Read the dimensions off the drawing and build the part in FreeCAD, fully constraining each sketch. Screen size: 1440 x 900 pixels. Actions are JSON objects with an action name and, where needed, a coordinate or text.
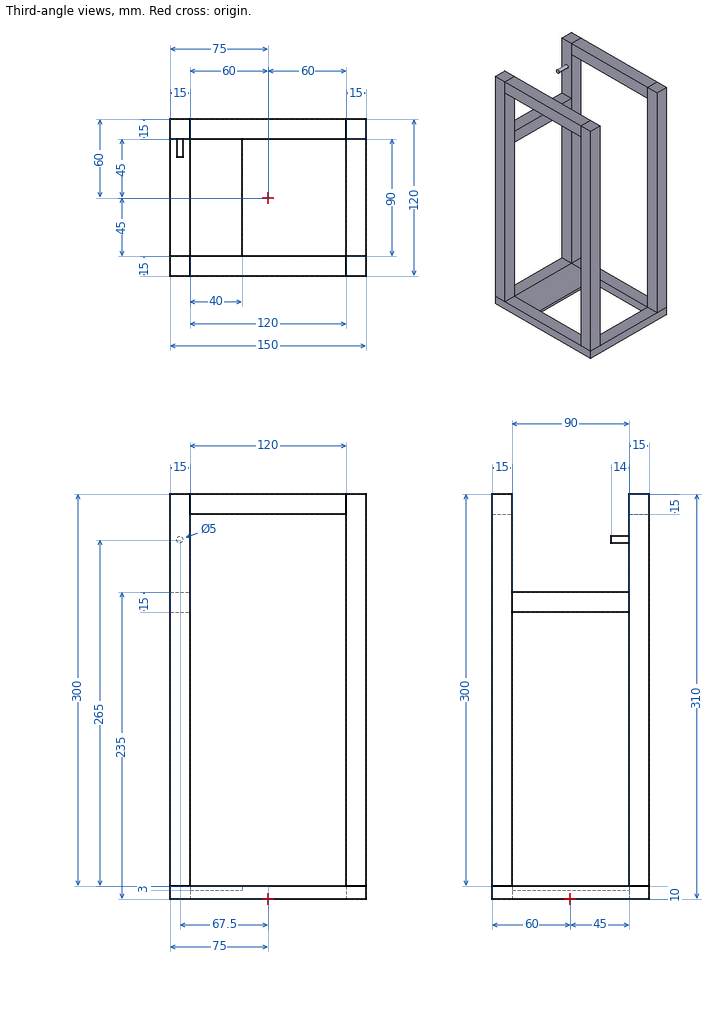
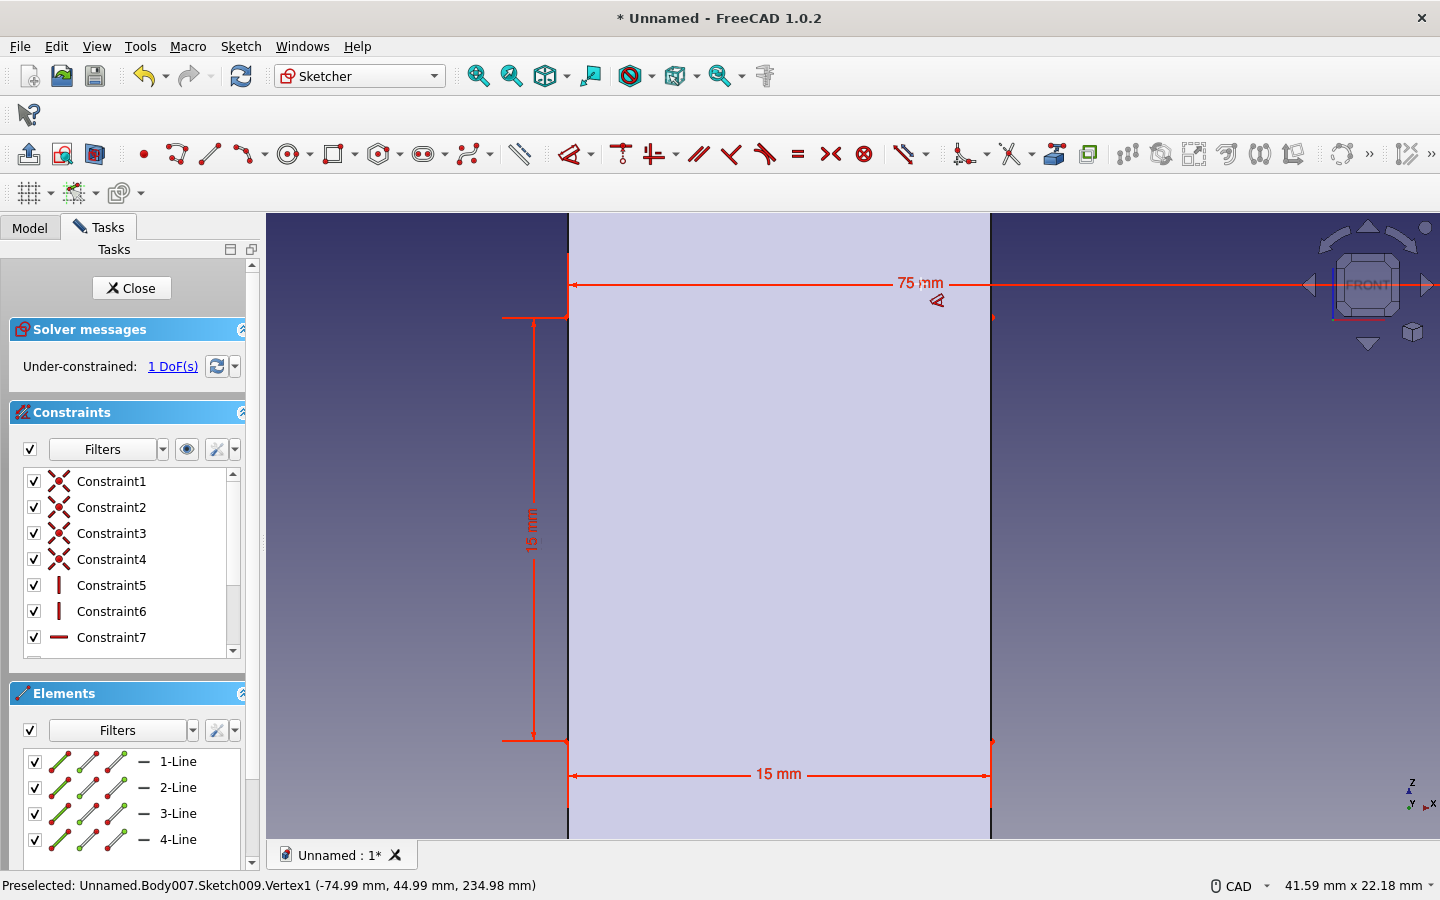
{"action": "left_click", "coordinate": [568, 318]}
{"action": "left_click", "coordinate": [534, 564]}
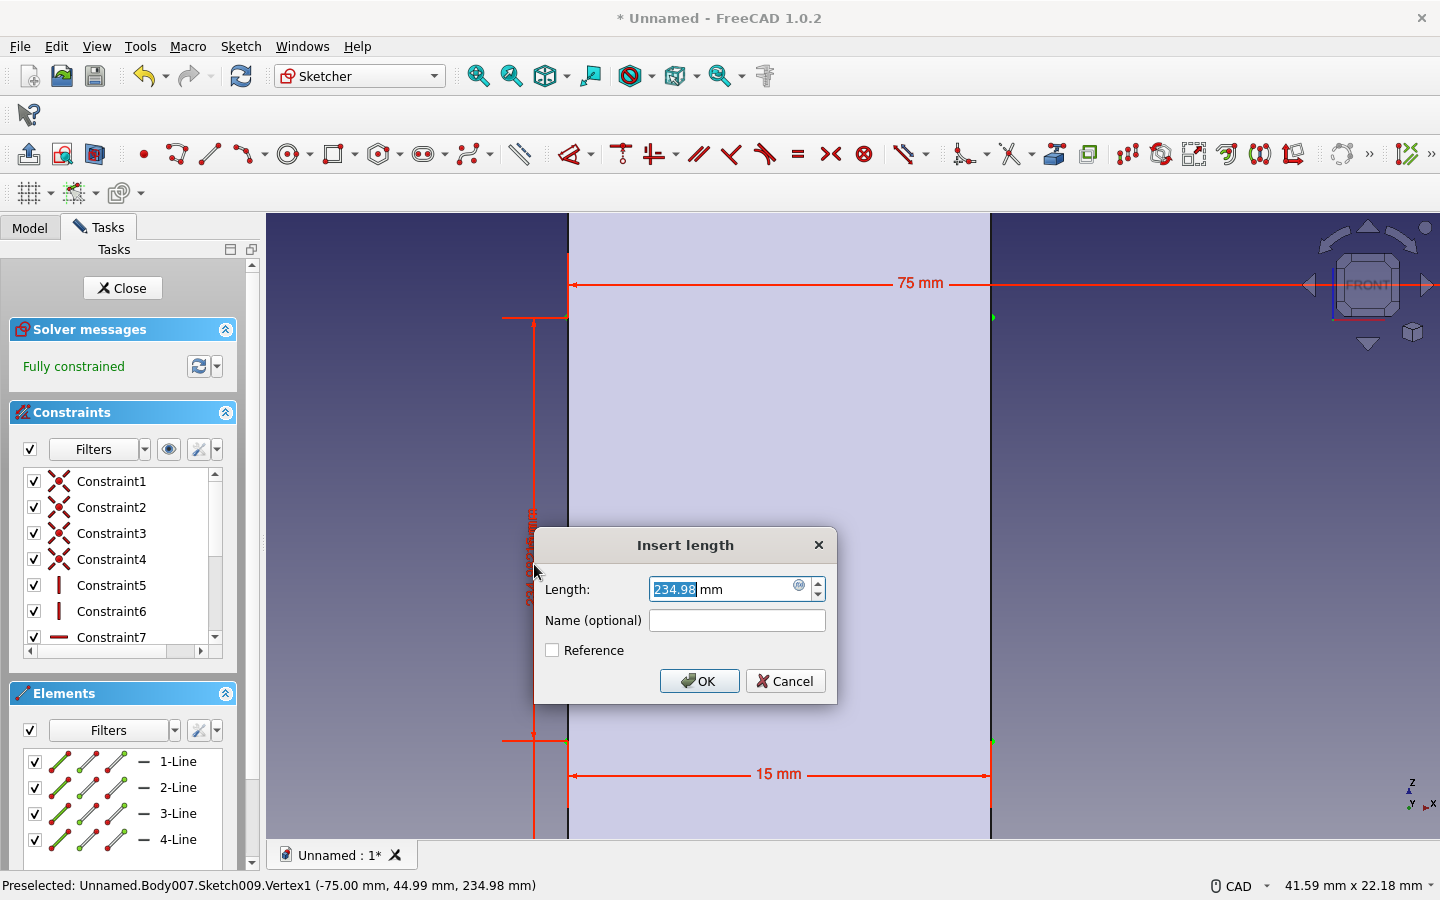
{"action": "type", "text": "235"}
{"action": "key", "text": "Return"}
{"action": "key", "text": "Escape"}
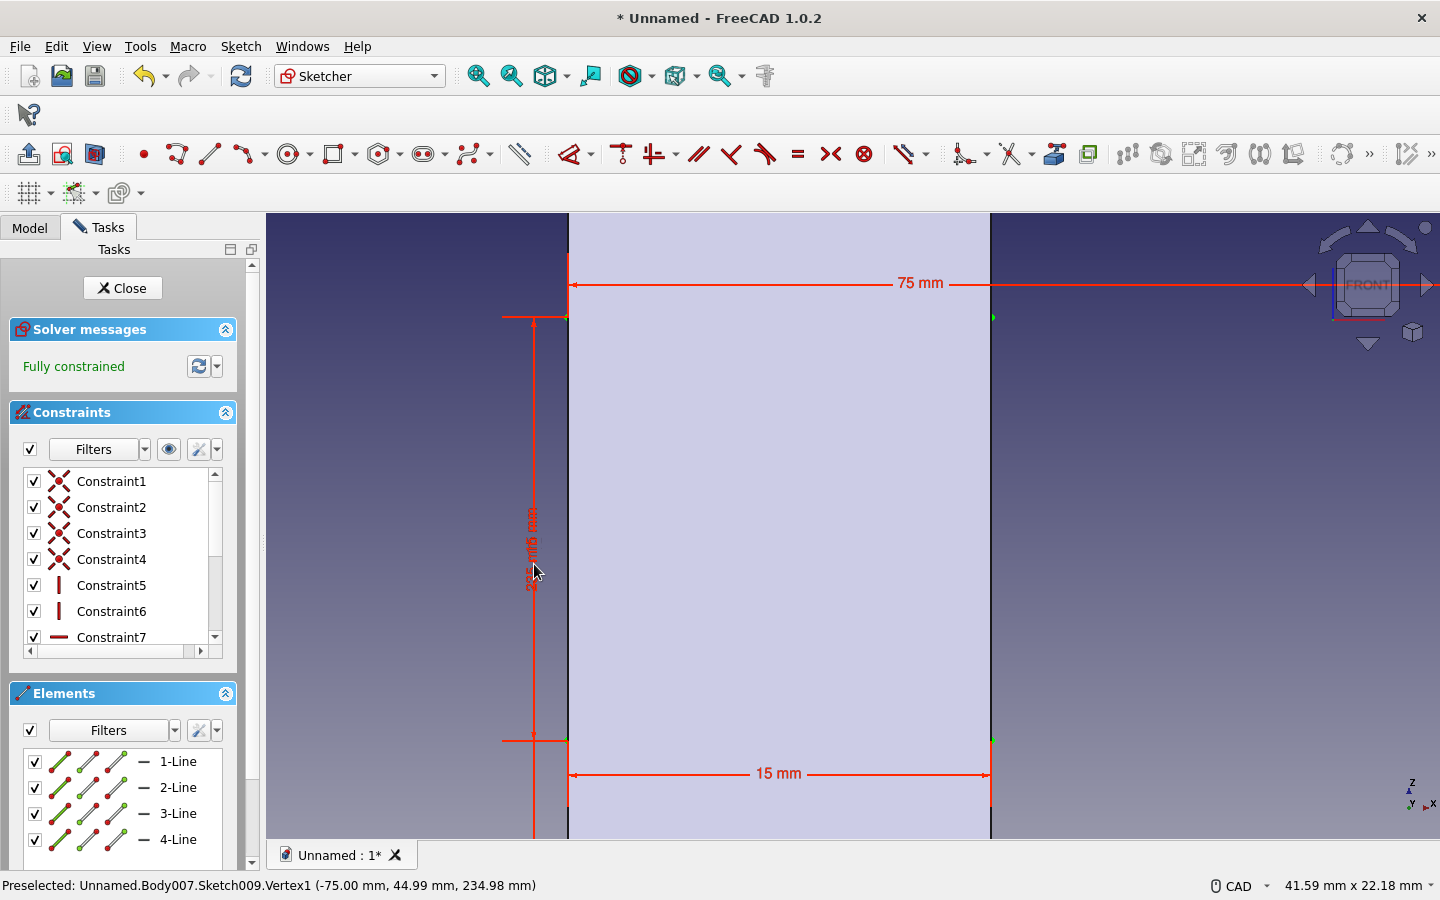
{"action": "left_click", "coordinate": [123, 288]}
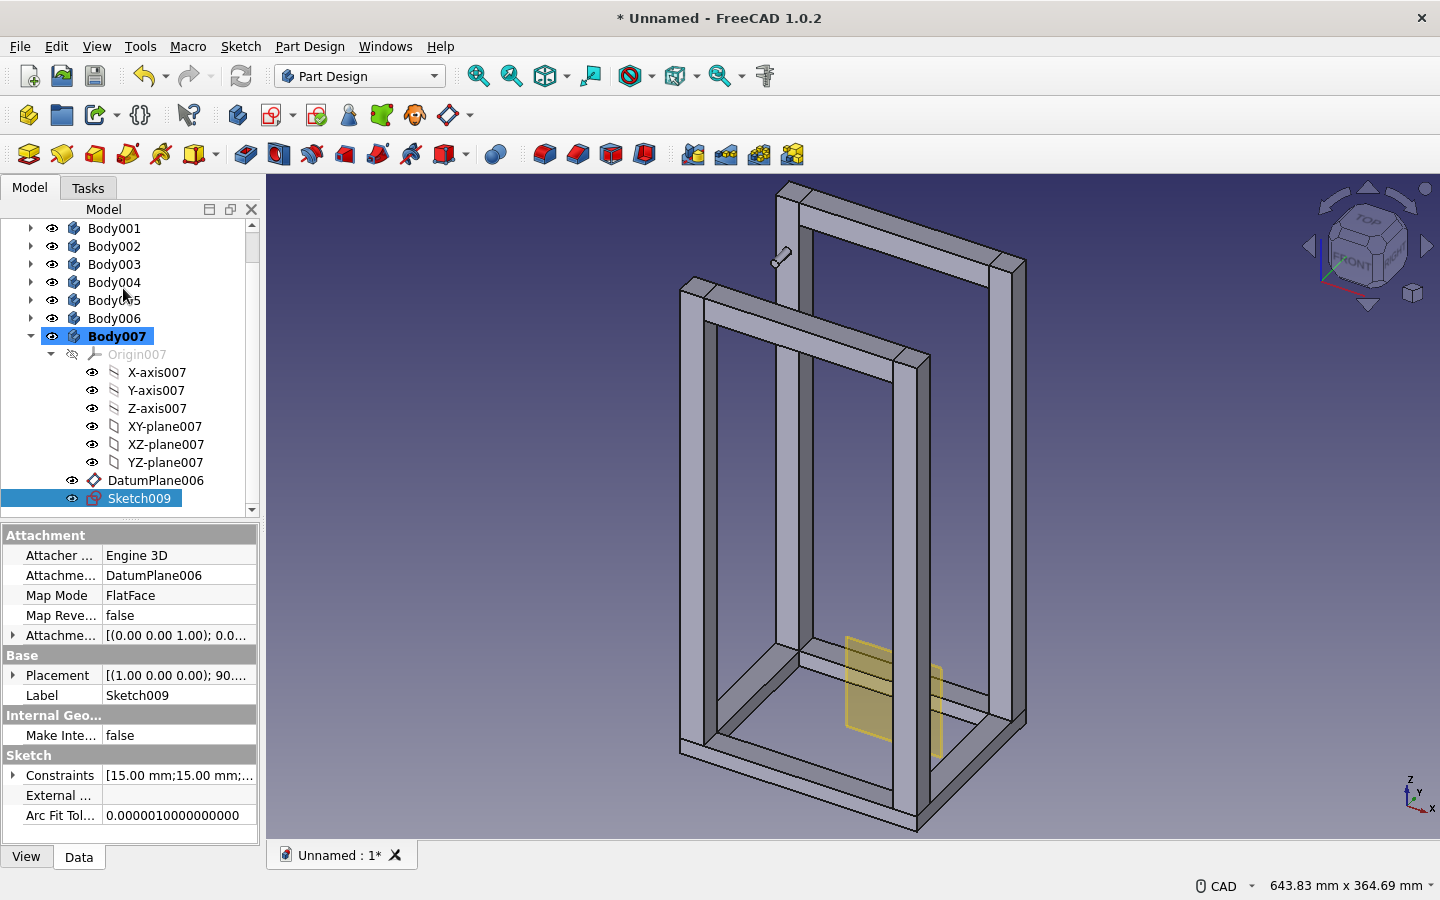
{"action": "left_click", "coordinate": [29, 154]}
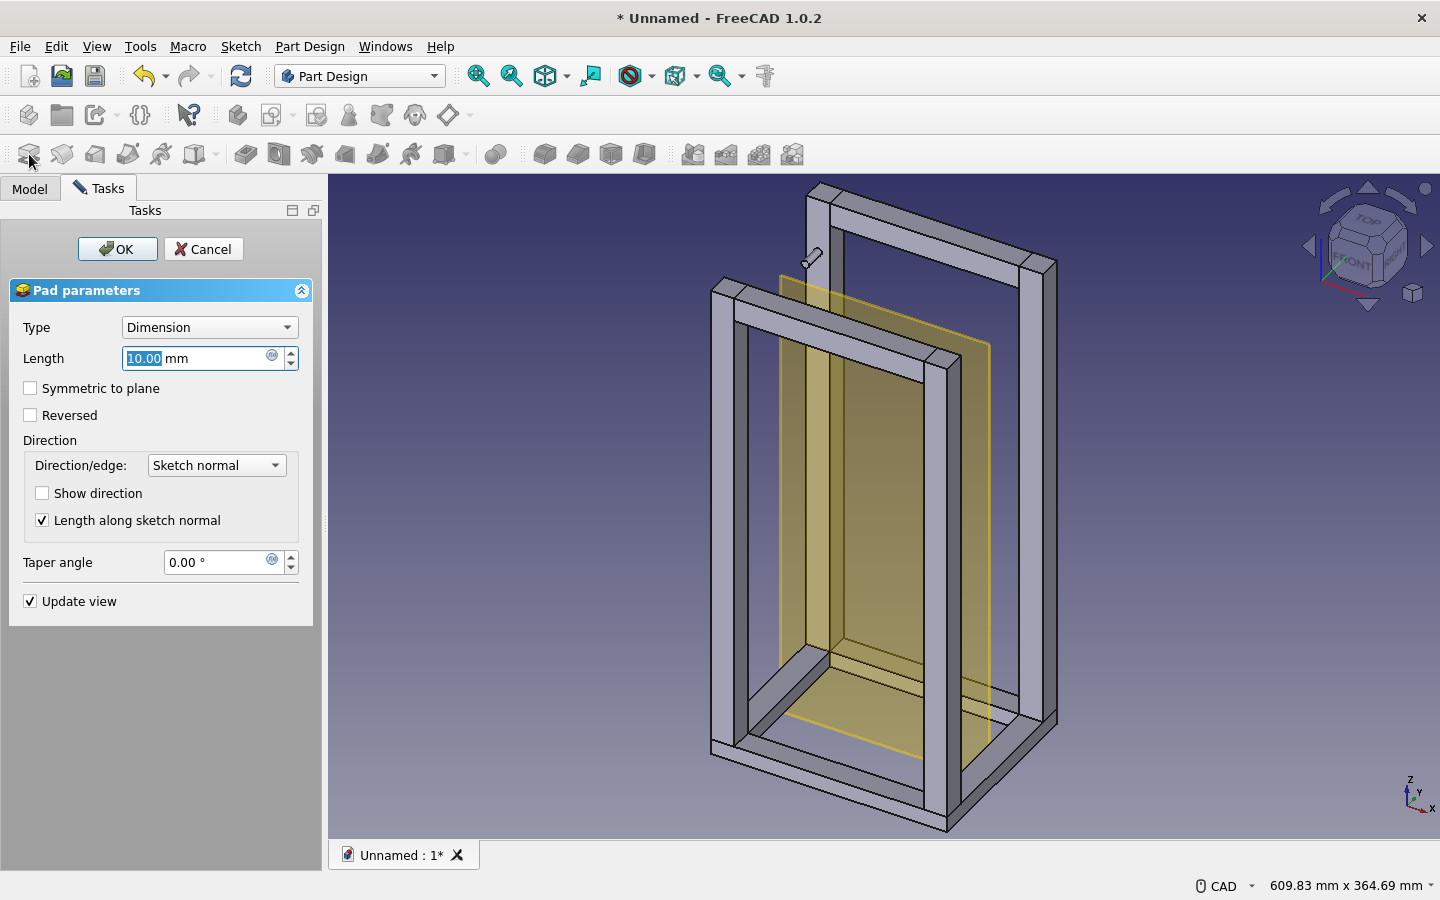
{"action": "type", "text": "90"}
{"action": "key", "text": "Tab"}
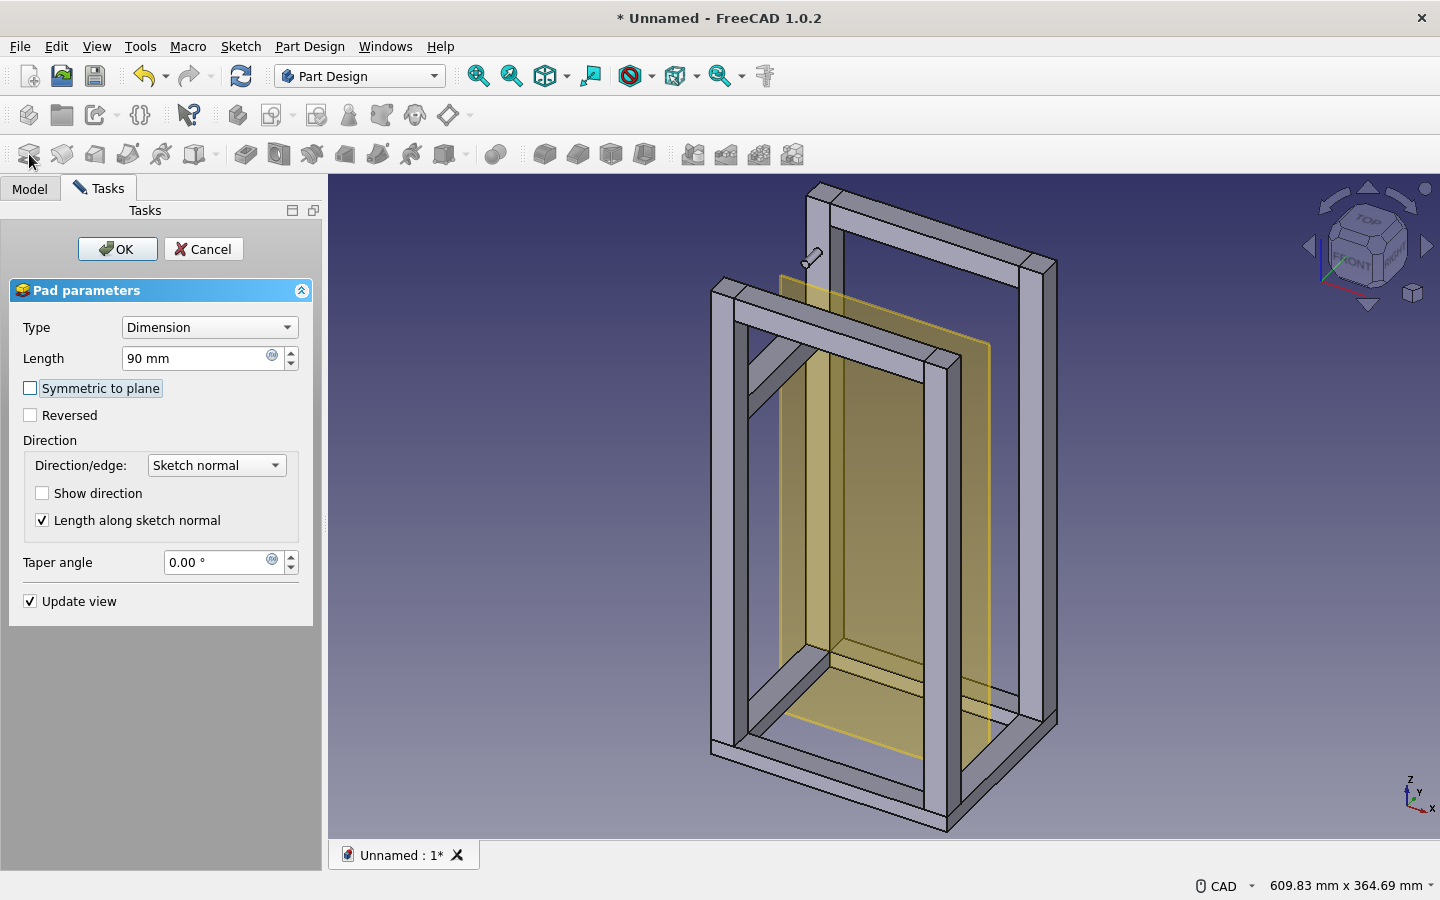
{"action": "left_click", "coordinate": [118, 249]}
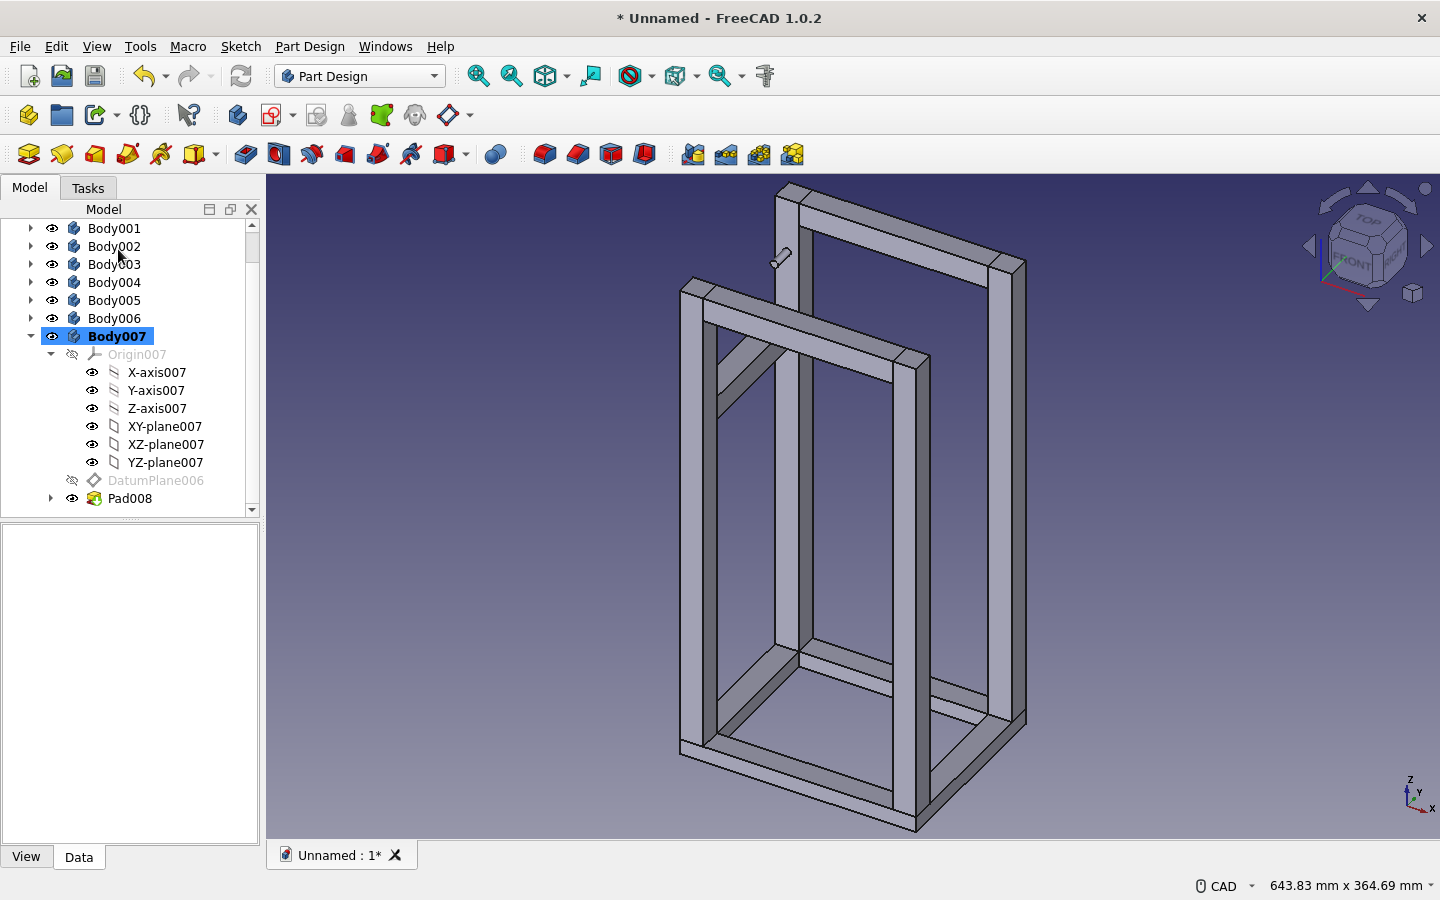
{"action": "left_click", "coordinate": [479, 76]}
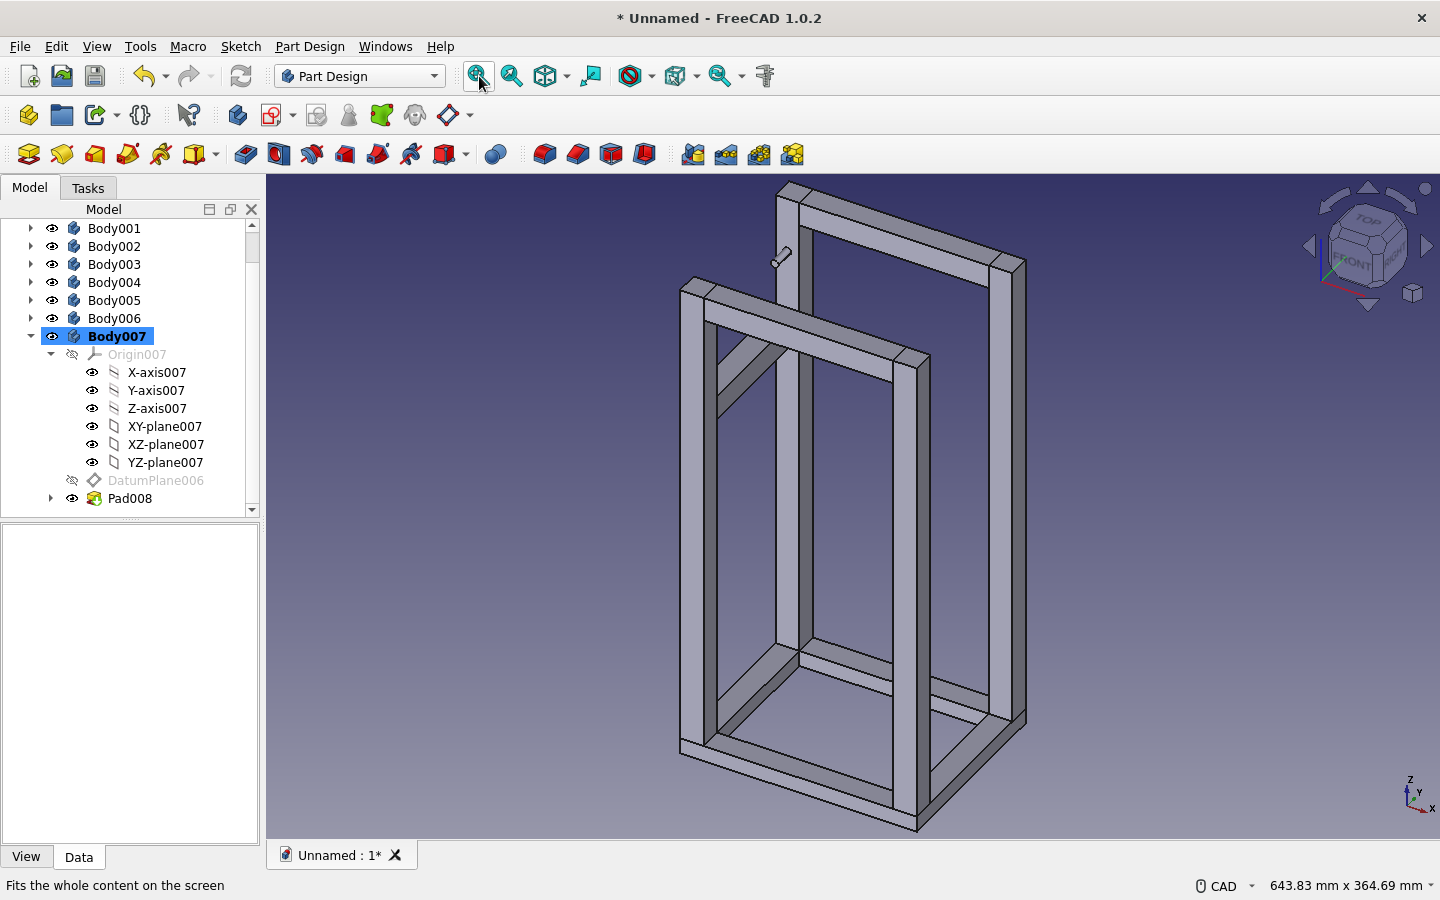
{"action": "left_click", "coordinate": [238, 116]}